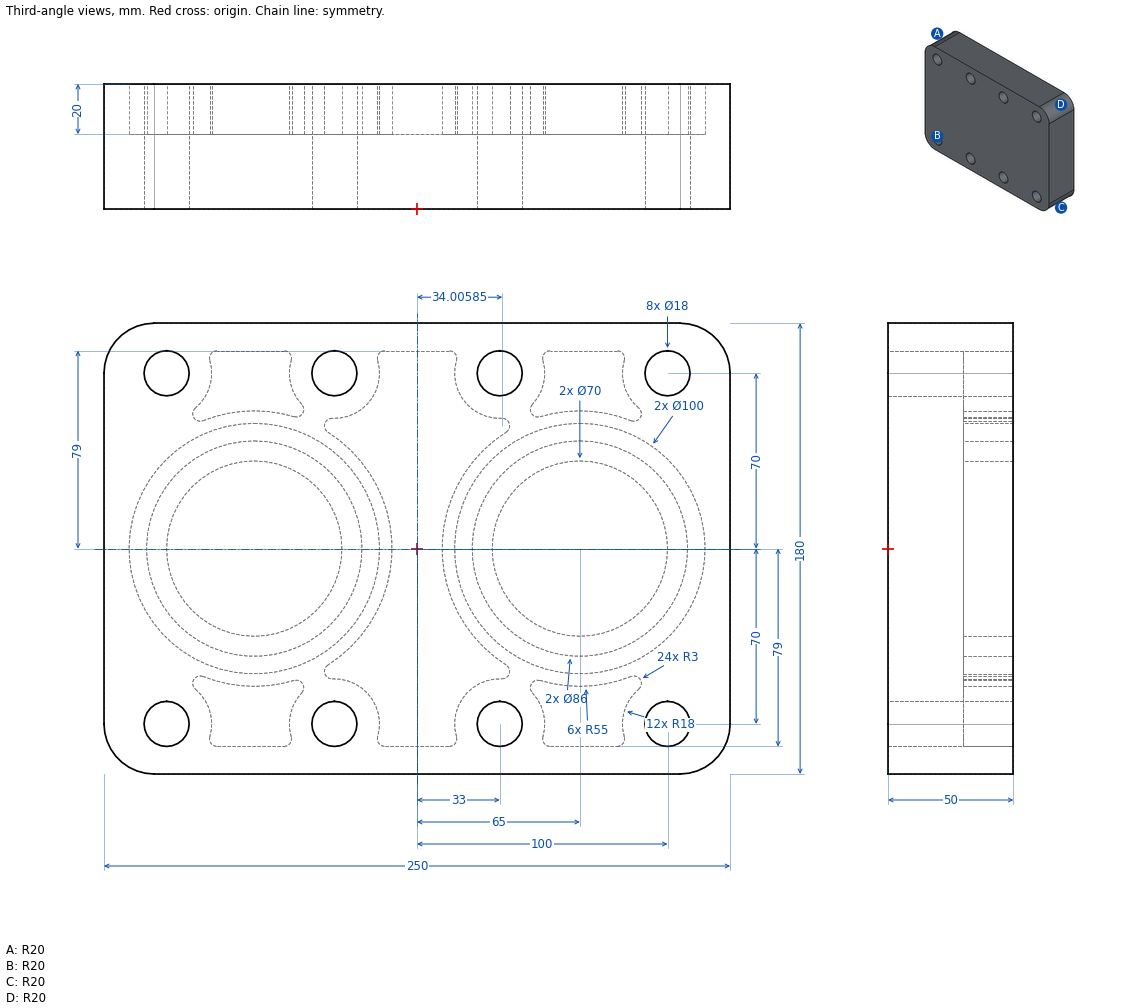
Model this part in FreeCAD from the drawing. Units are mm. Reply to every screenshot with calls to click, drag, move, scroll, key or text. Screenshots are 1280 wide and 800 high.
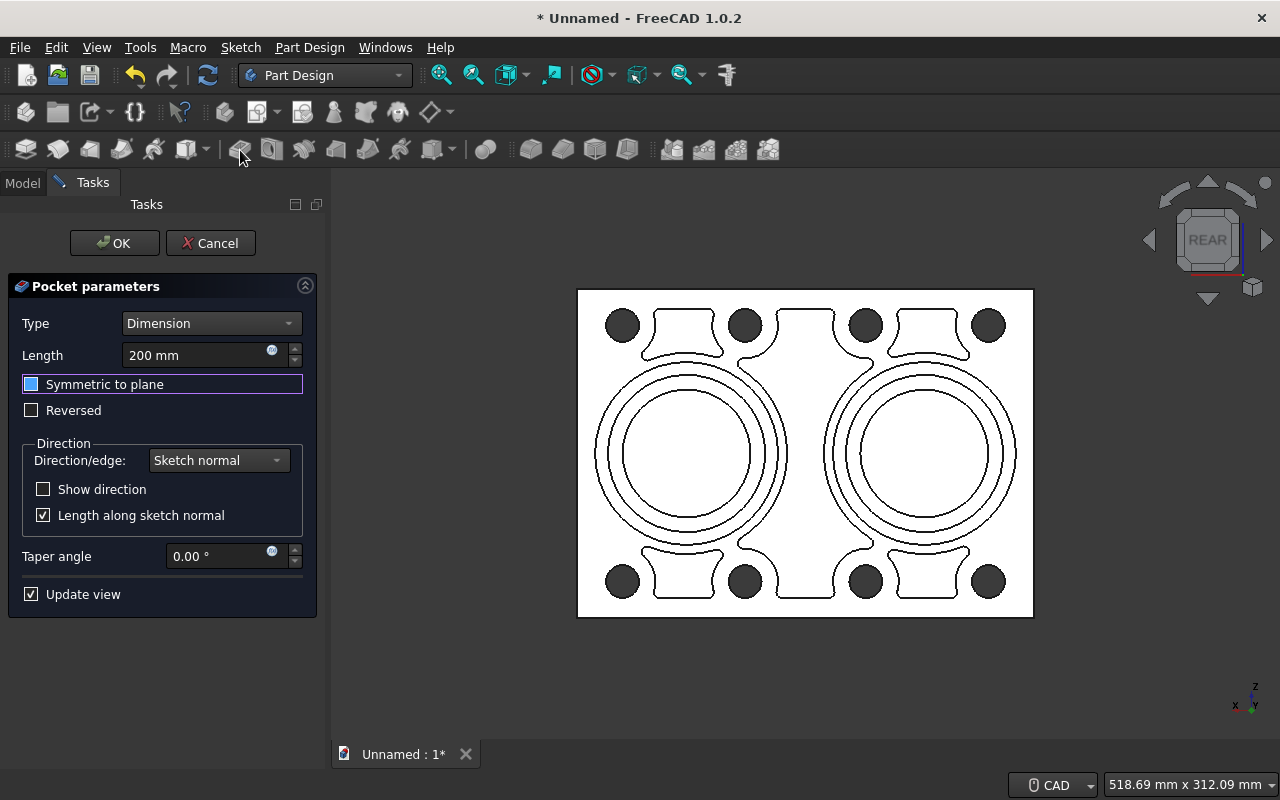
click(115, 243)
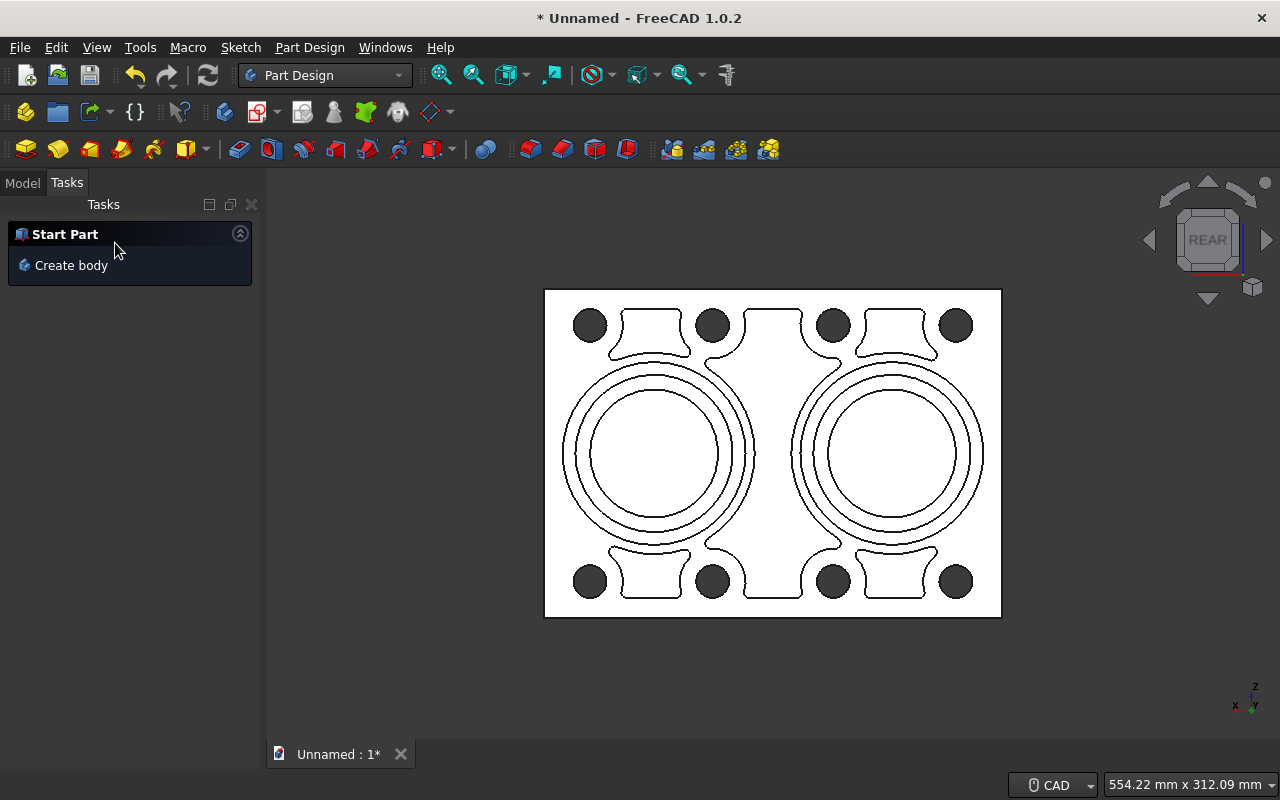
key(0)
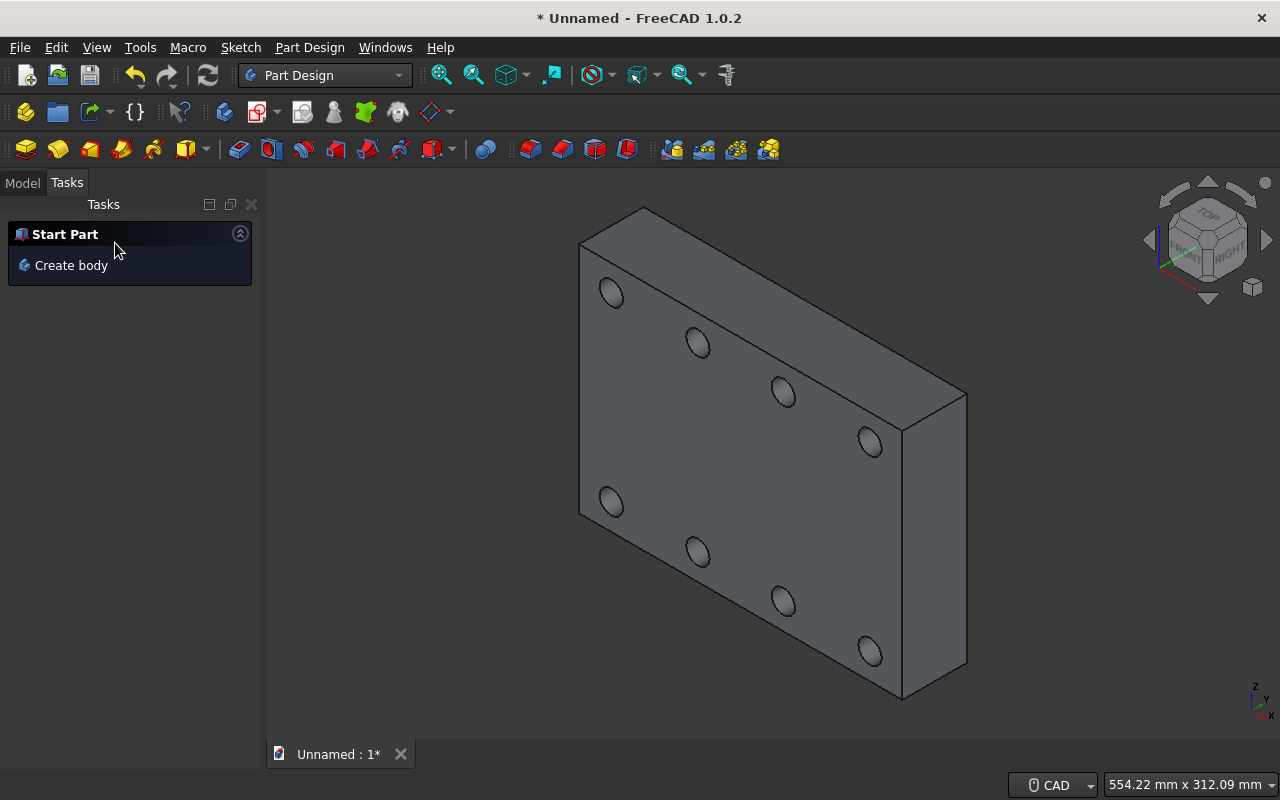
key(2)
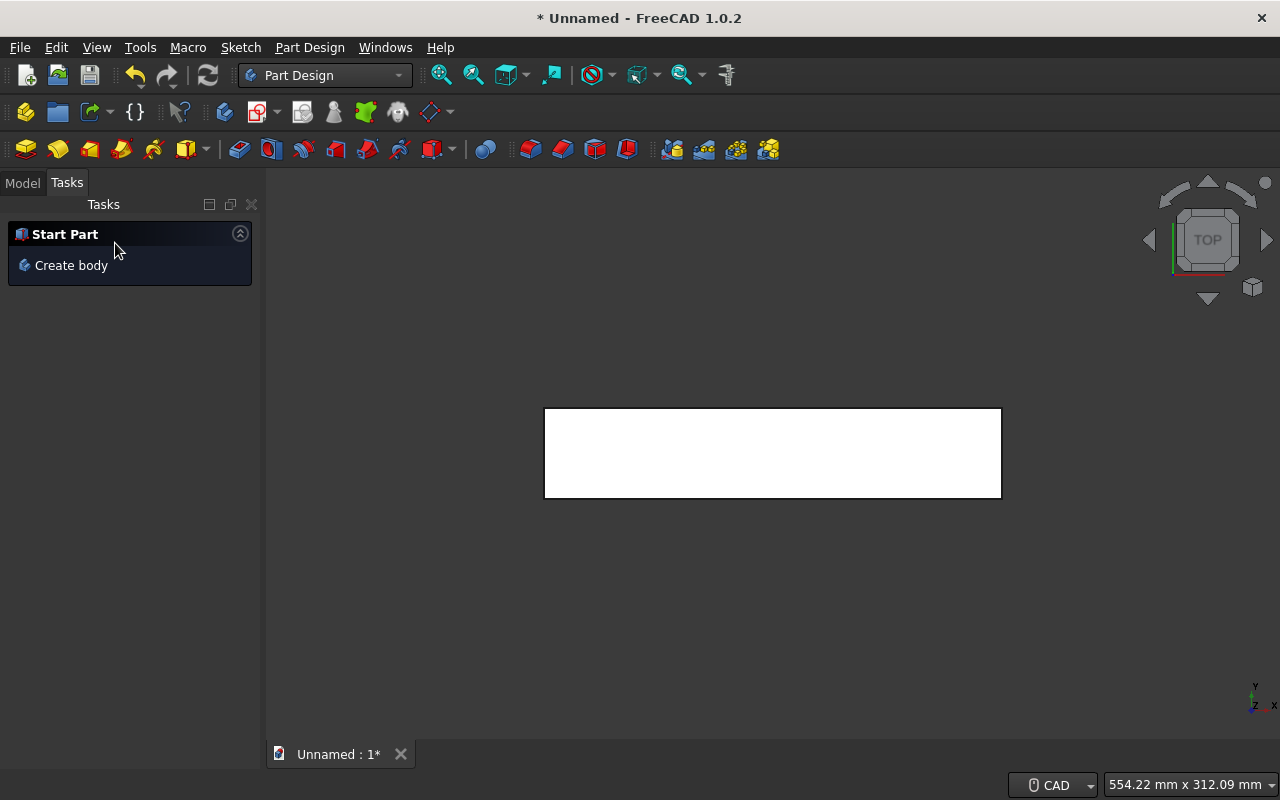
click(544, 452)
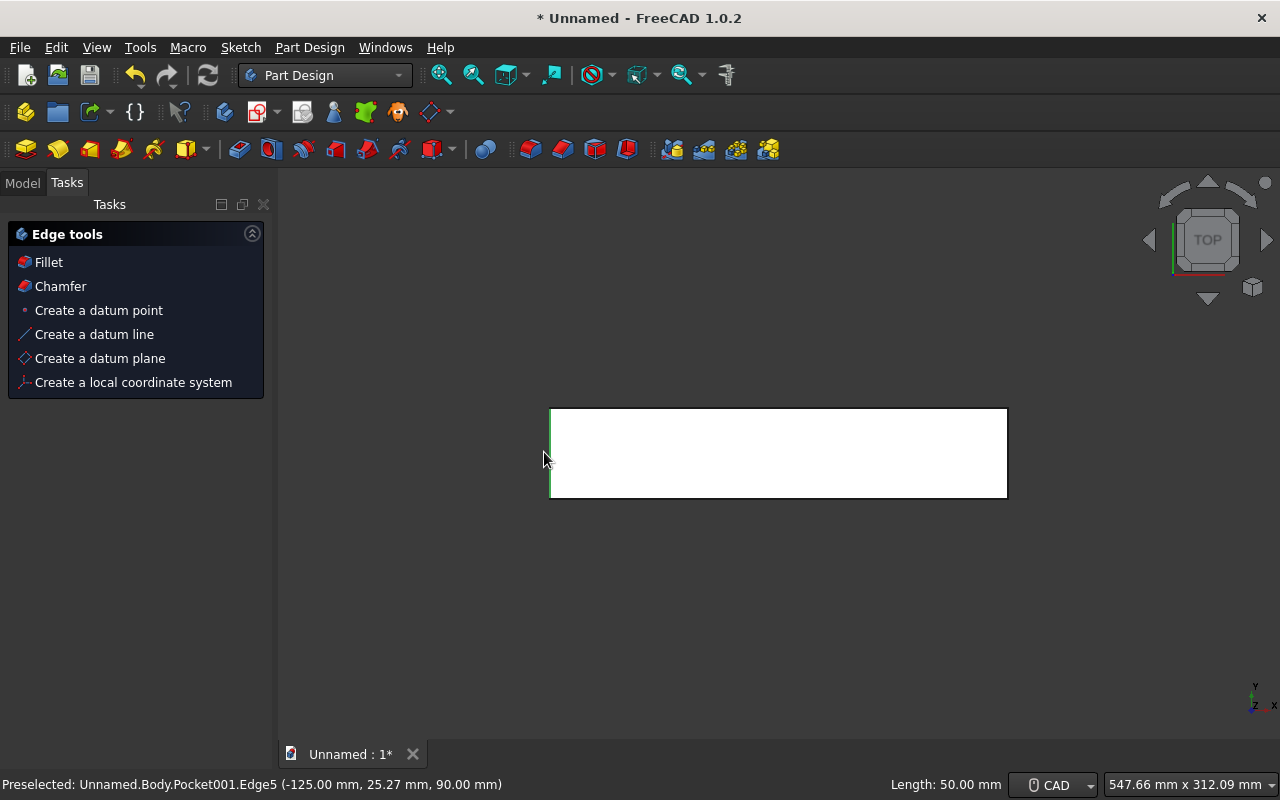
click(532, 150)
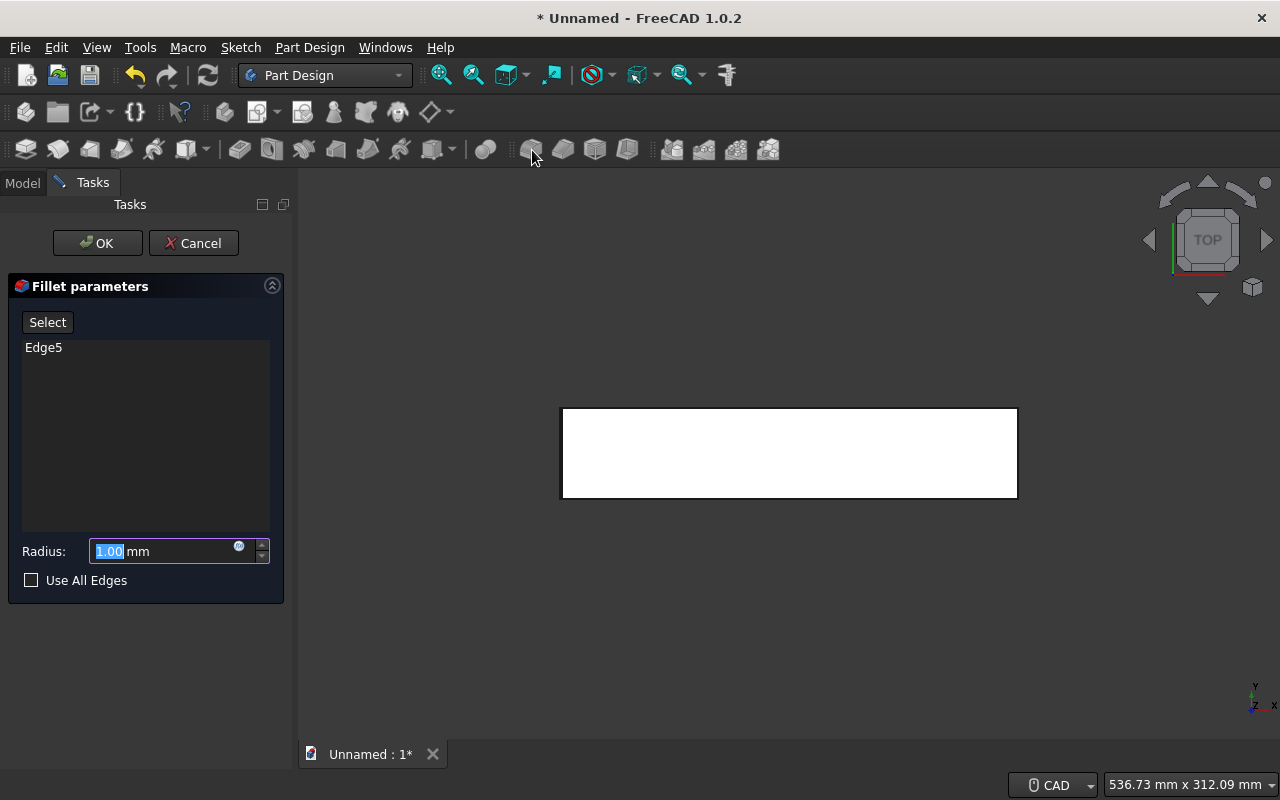
text(20)
key(Tab)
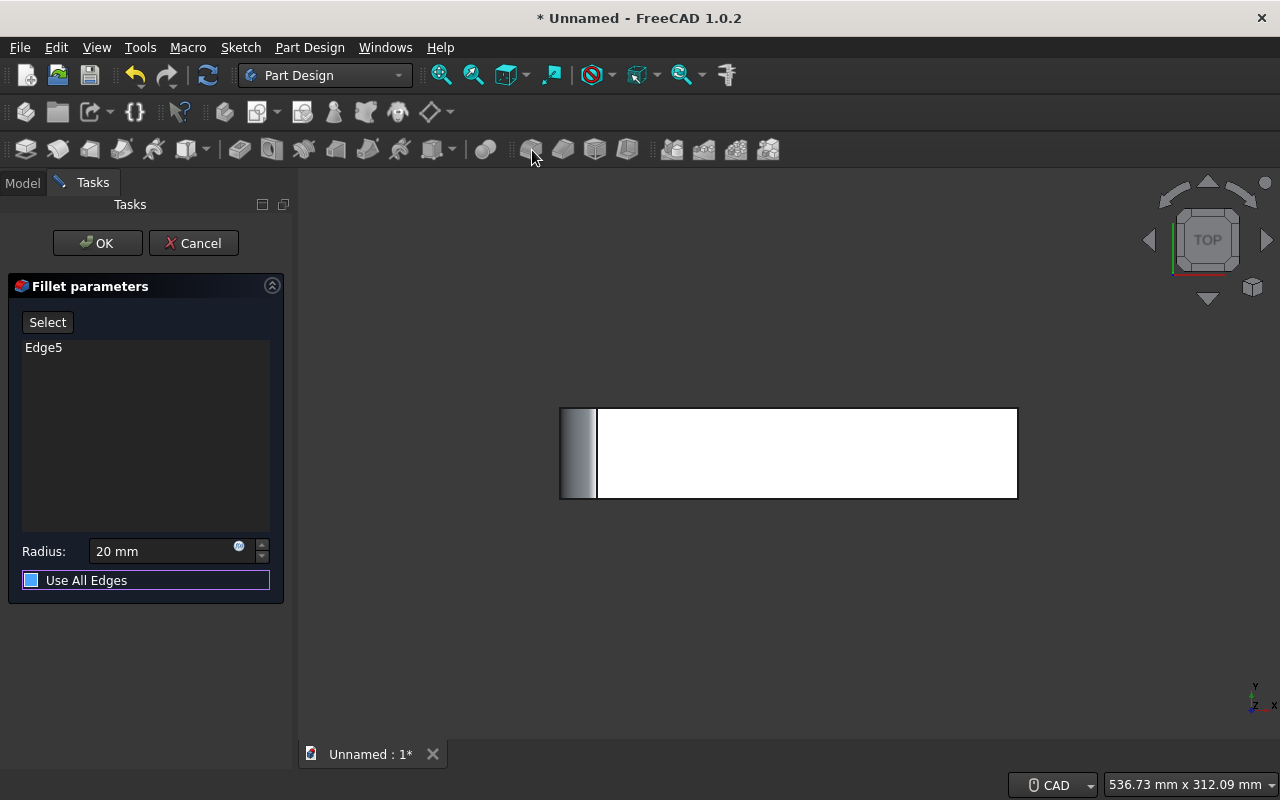
click(98, 243)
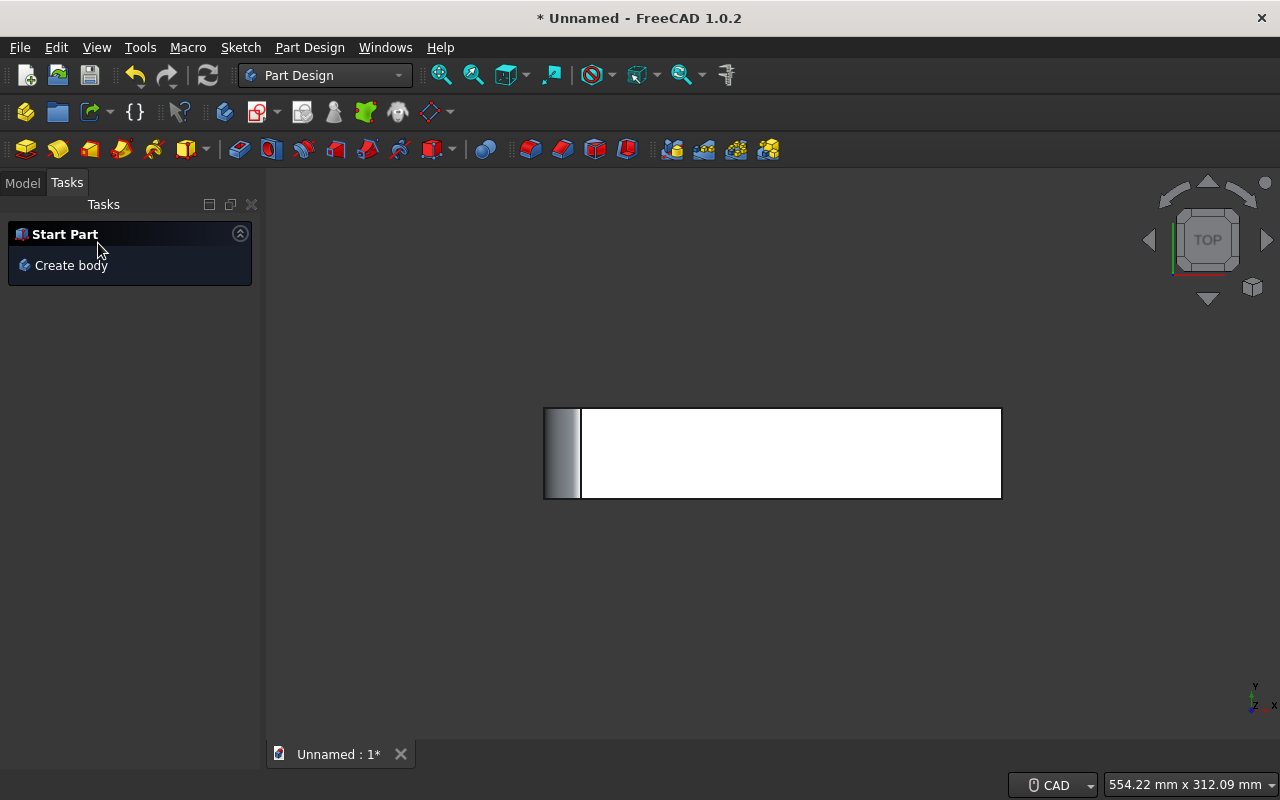
key(0)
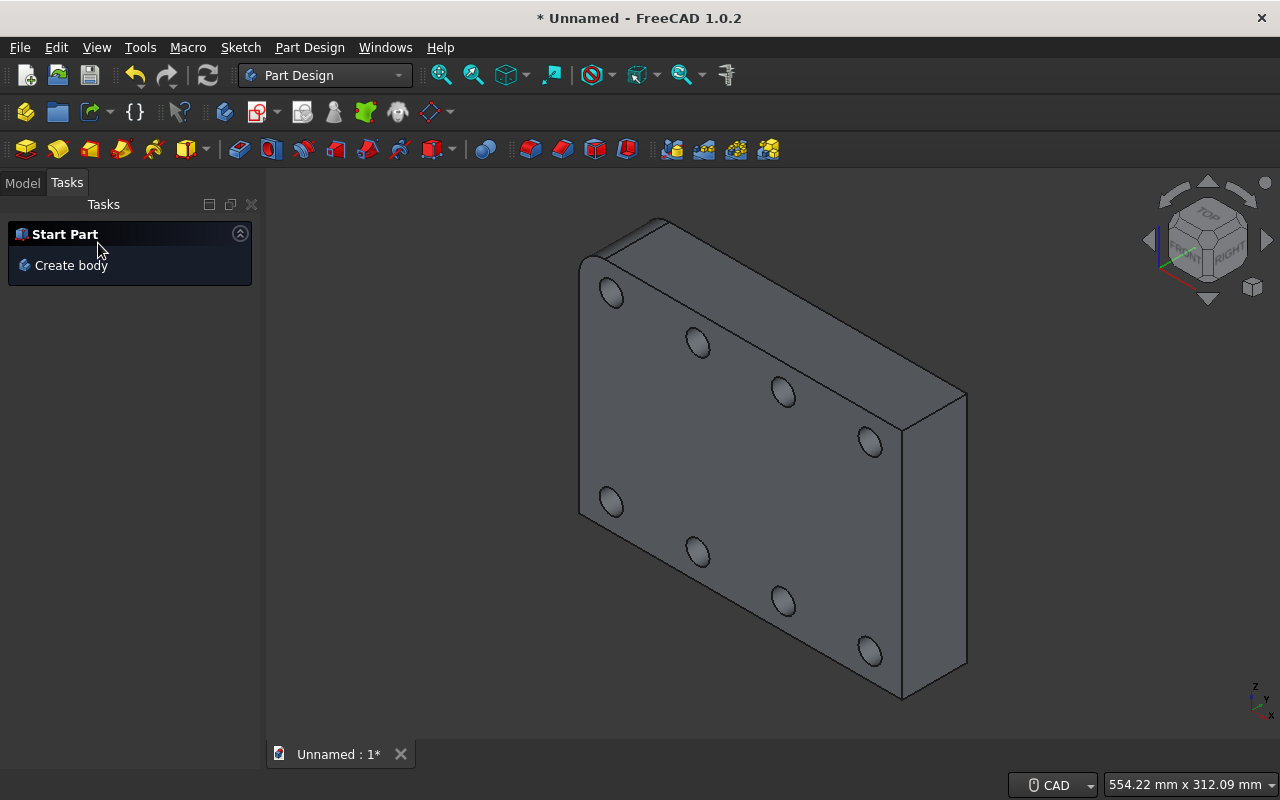
key(2)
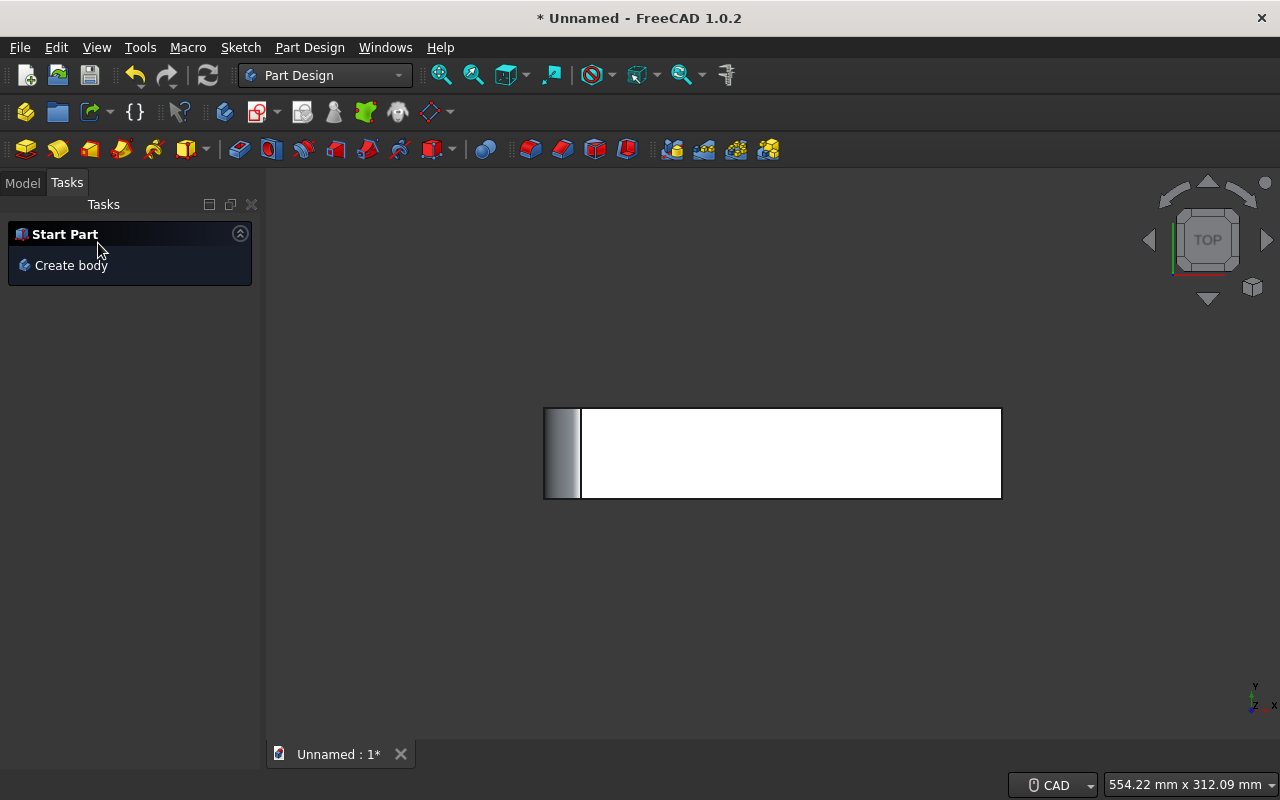
key(1)